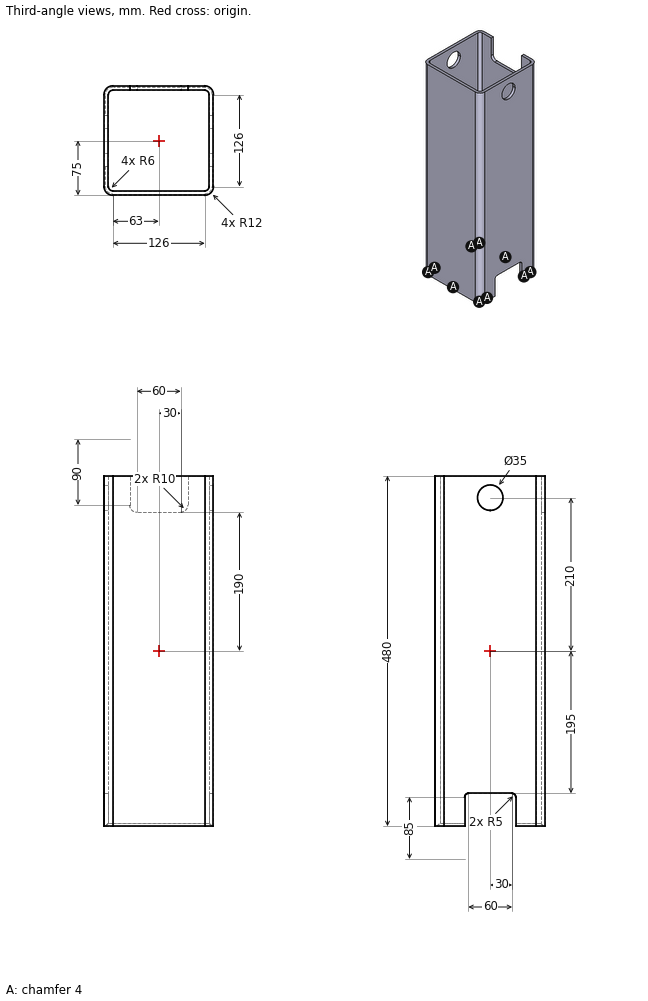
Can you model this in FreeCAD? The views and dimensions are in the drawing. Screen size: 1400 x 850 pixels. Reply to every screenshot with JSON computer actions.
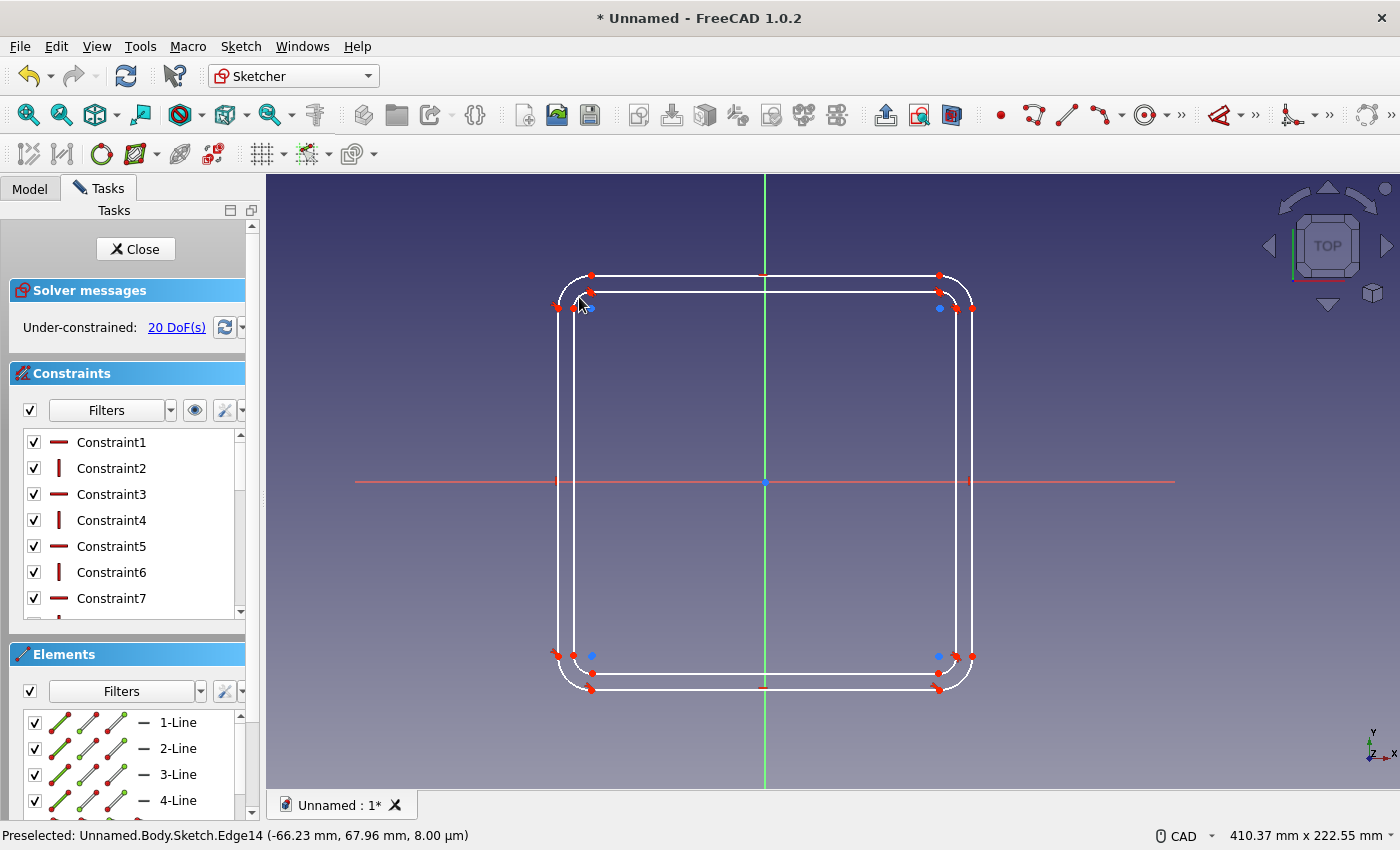
{"action": "left_click", "coordinate": [695, 292]}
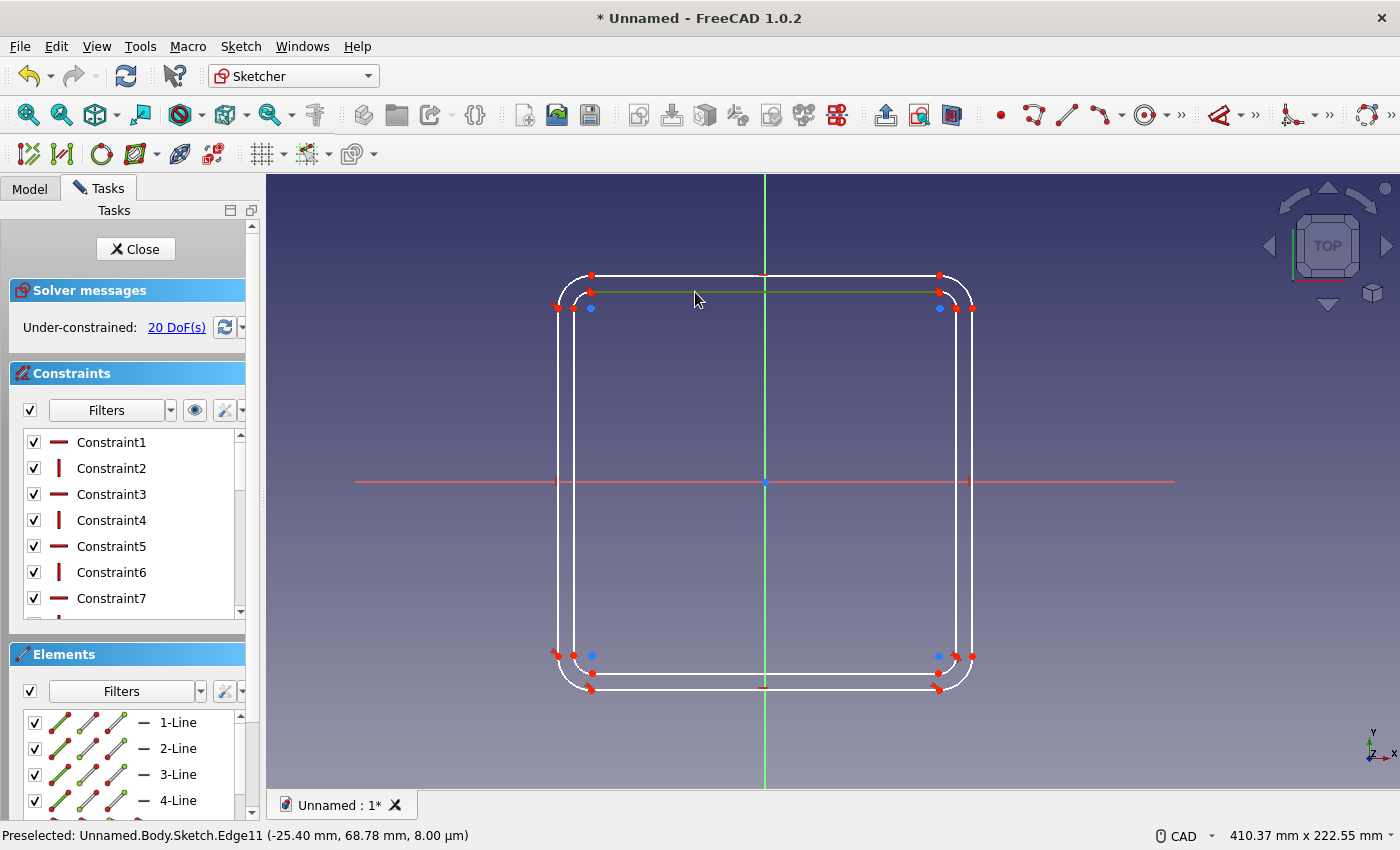
{"action": "left_click", "coordinate": [579, 297]}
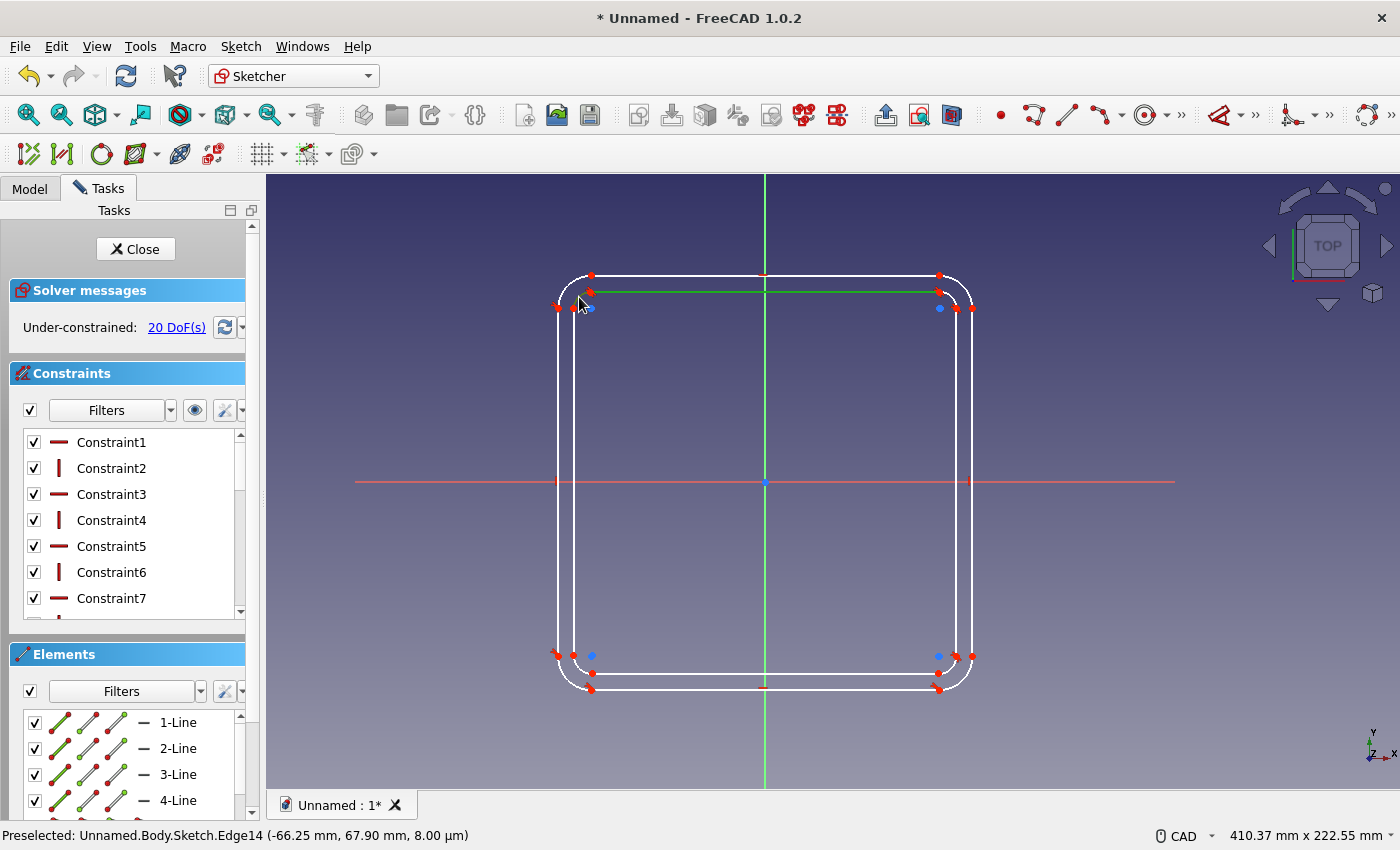
{"action": "key", "text": "t"}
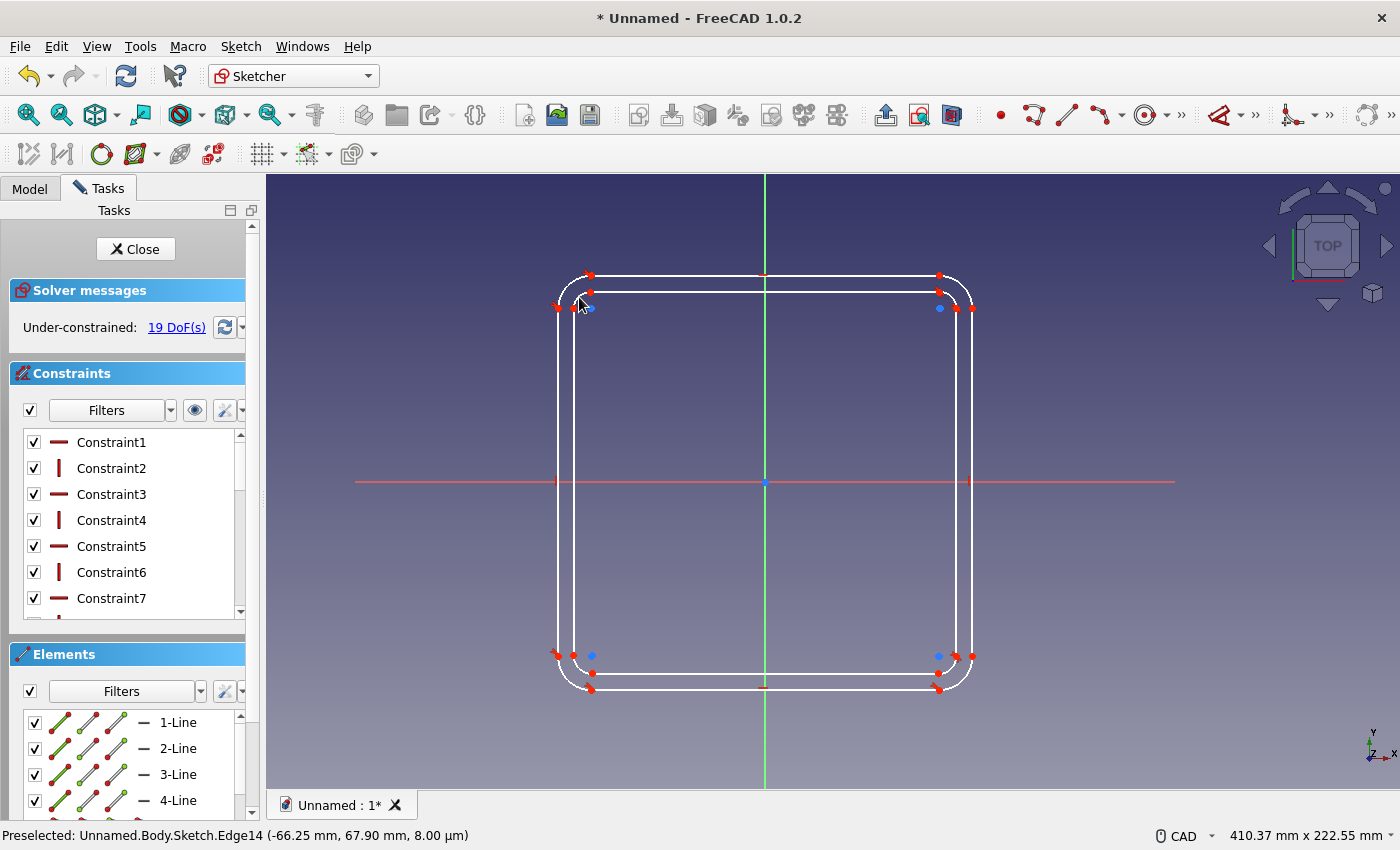
{"action": "left_click", "coordinate": [695, 292]}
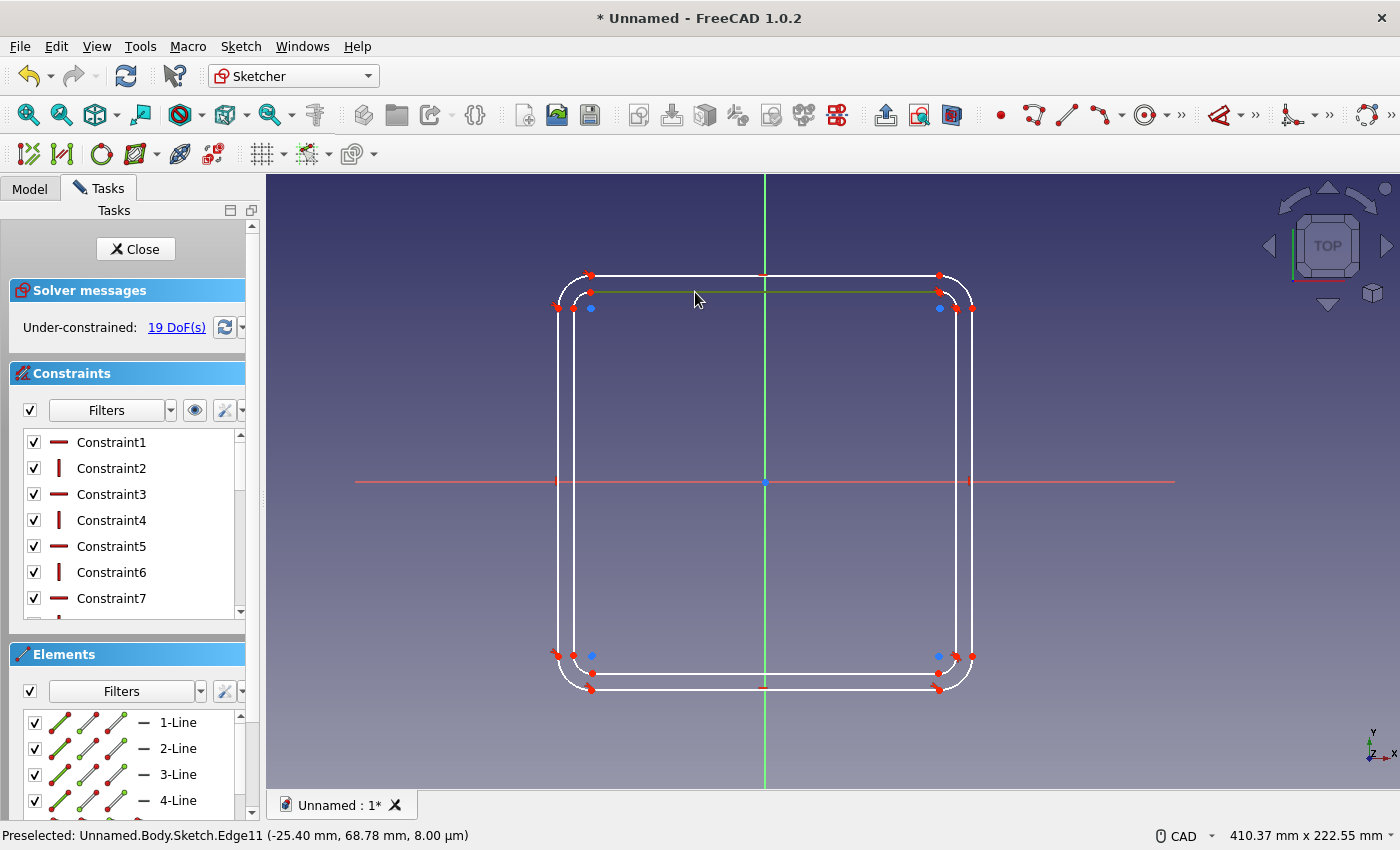
{"action": "left_click", "coordinate": [952, 297]}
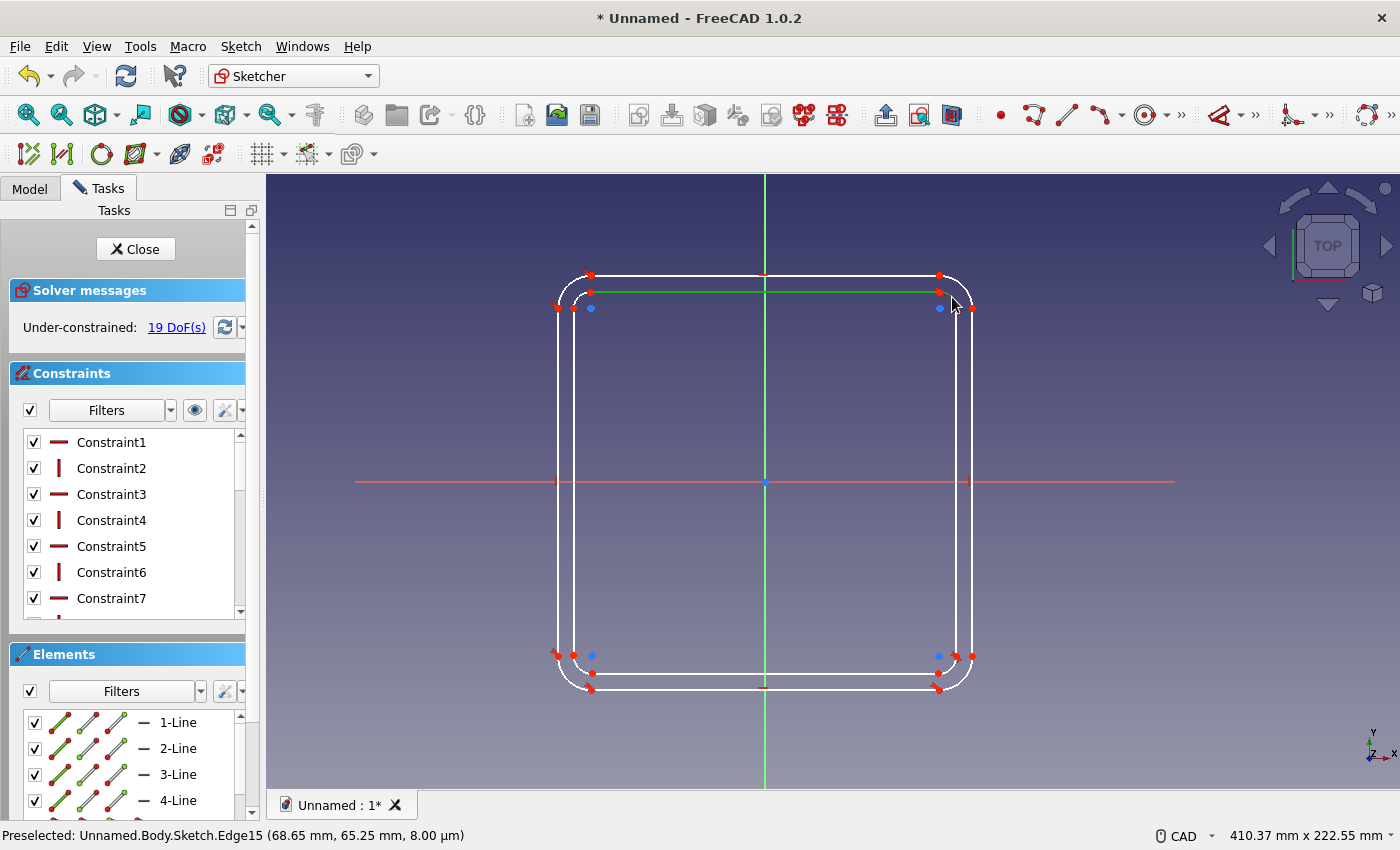
{"action": "key", "text": "t"}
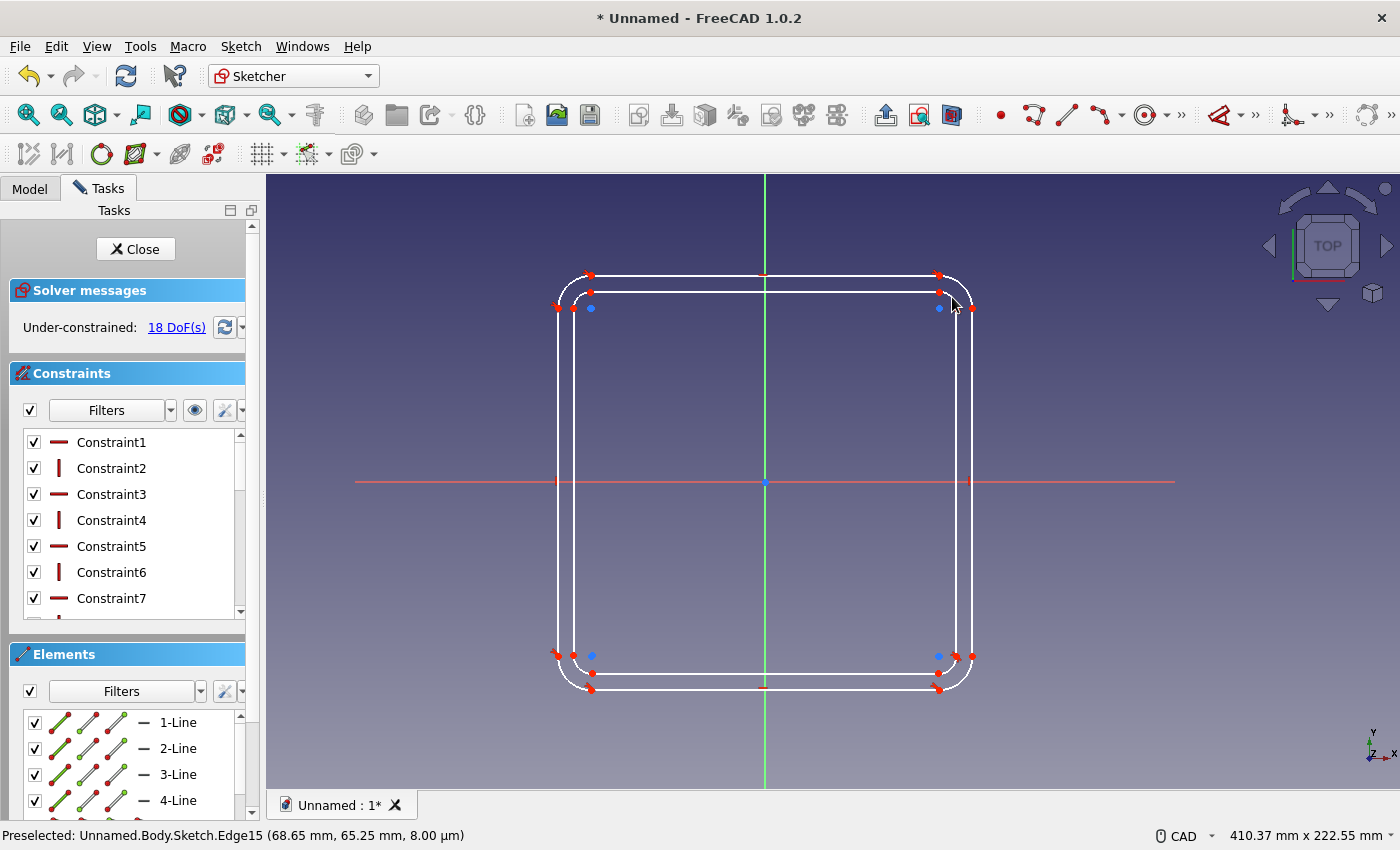
{"action": "left_click", "coordinate": [956, 413]}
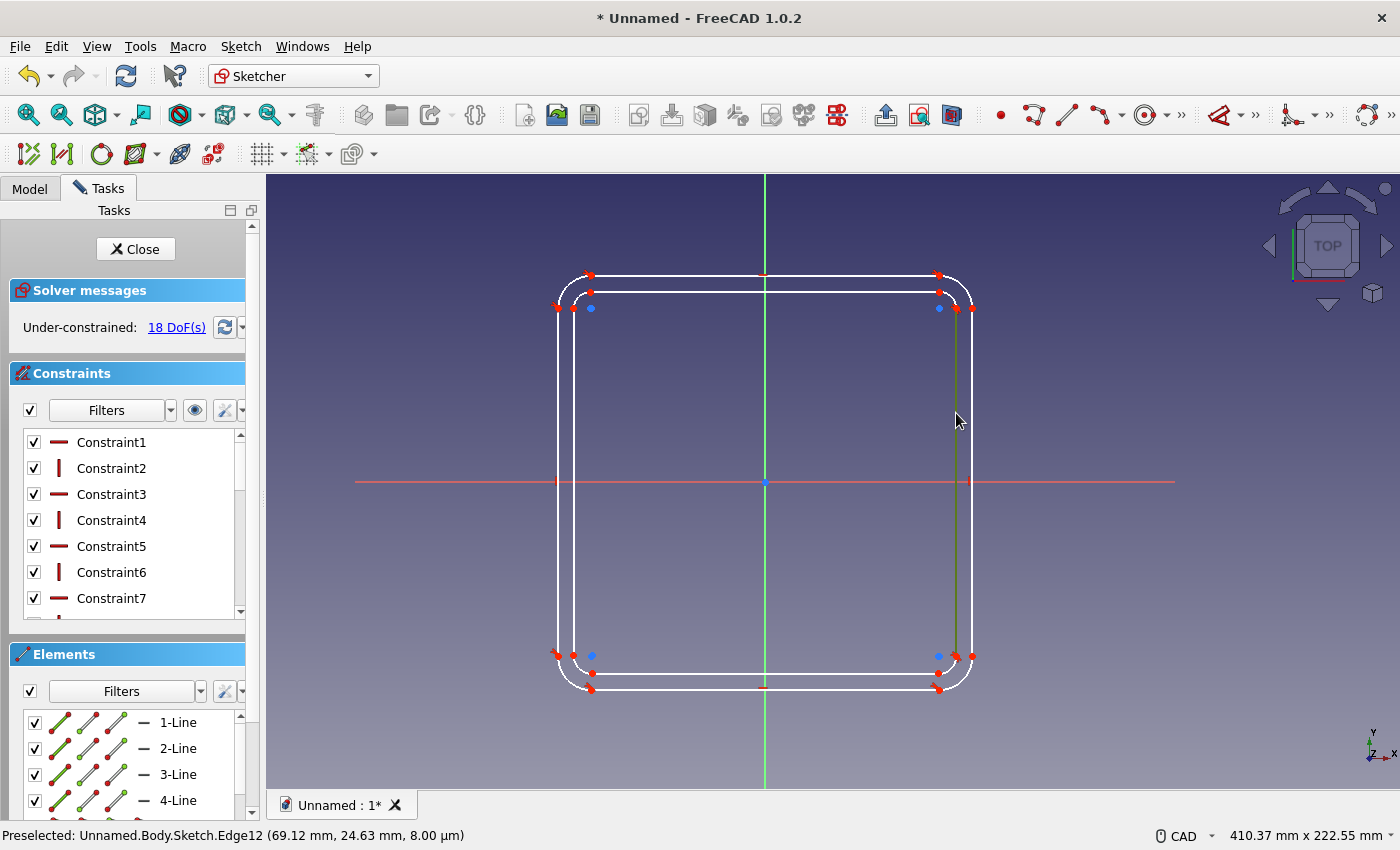
{"action": "left_click", "coordinate": [952, 297]}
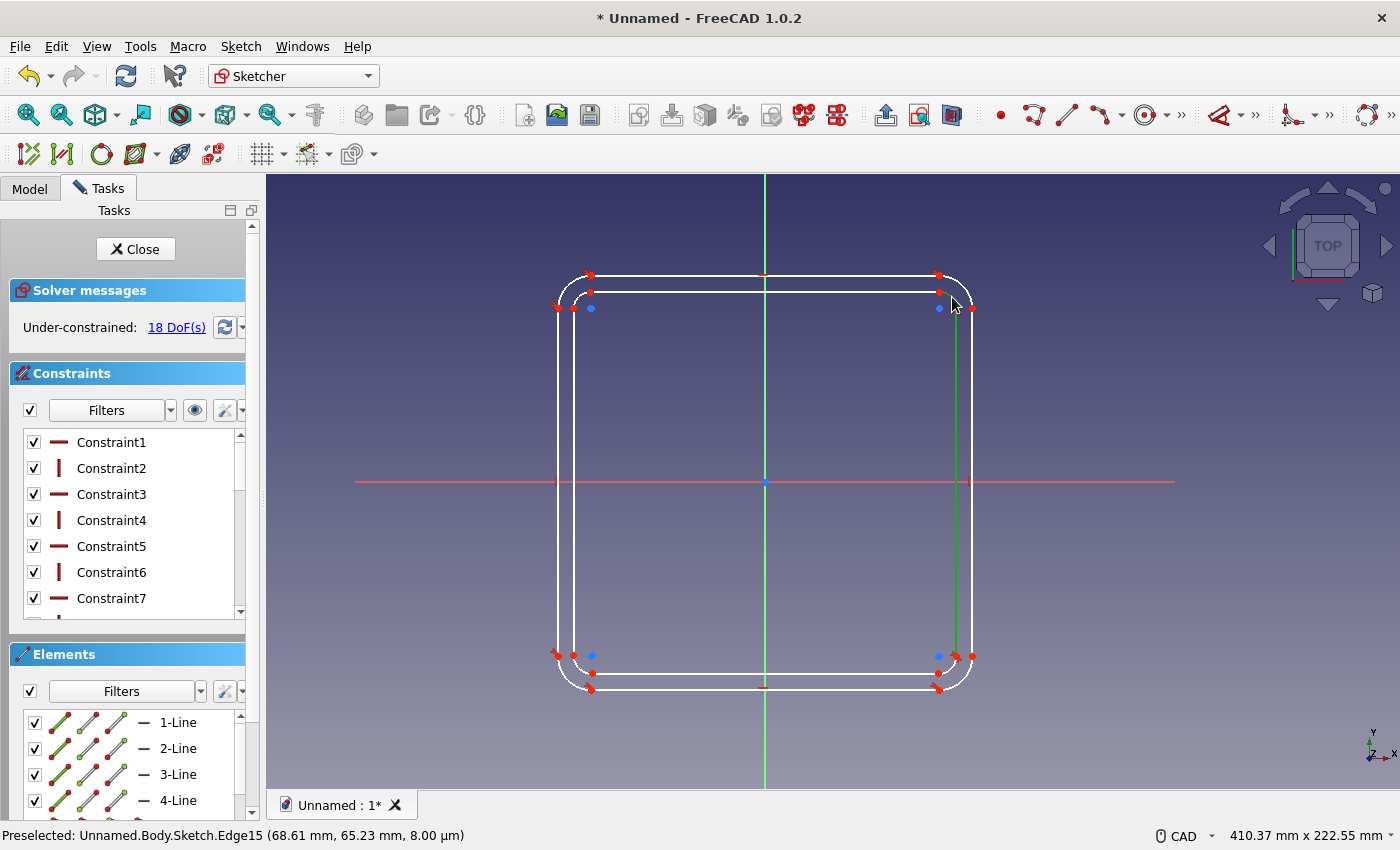
{"action": "key", "text": "t"}